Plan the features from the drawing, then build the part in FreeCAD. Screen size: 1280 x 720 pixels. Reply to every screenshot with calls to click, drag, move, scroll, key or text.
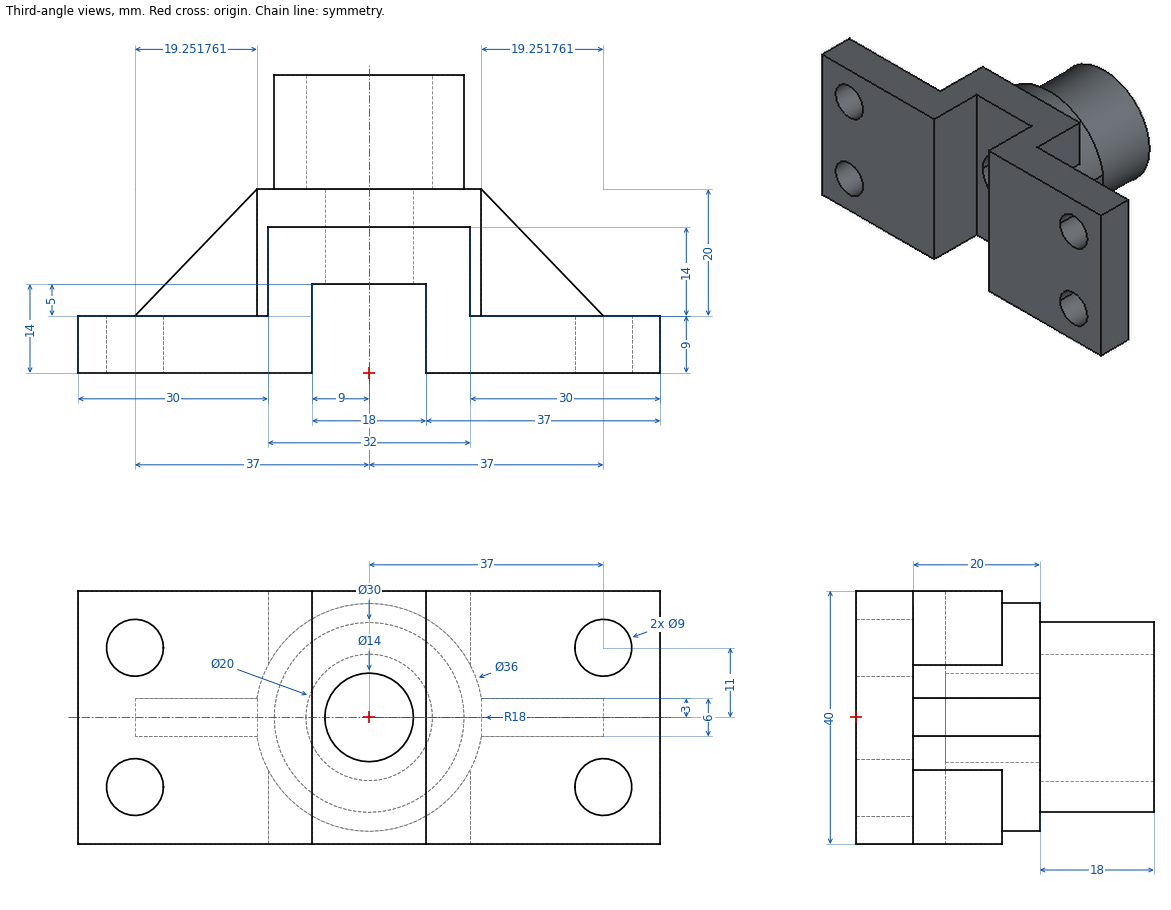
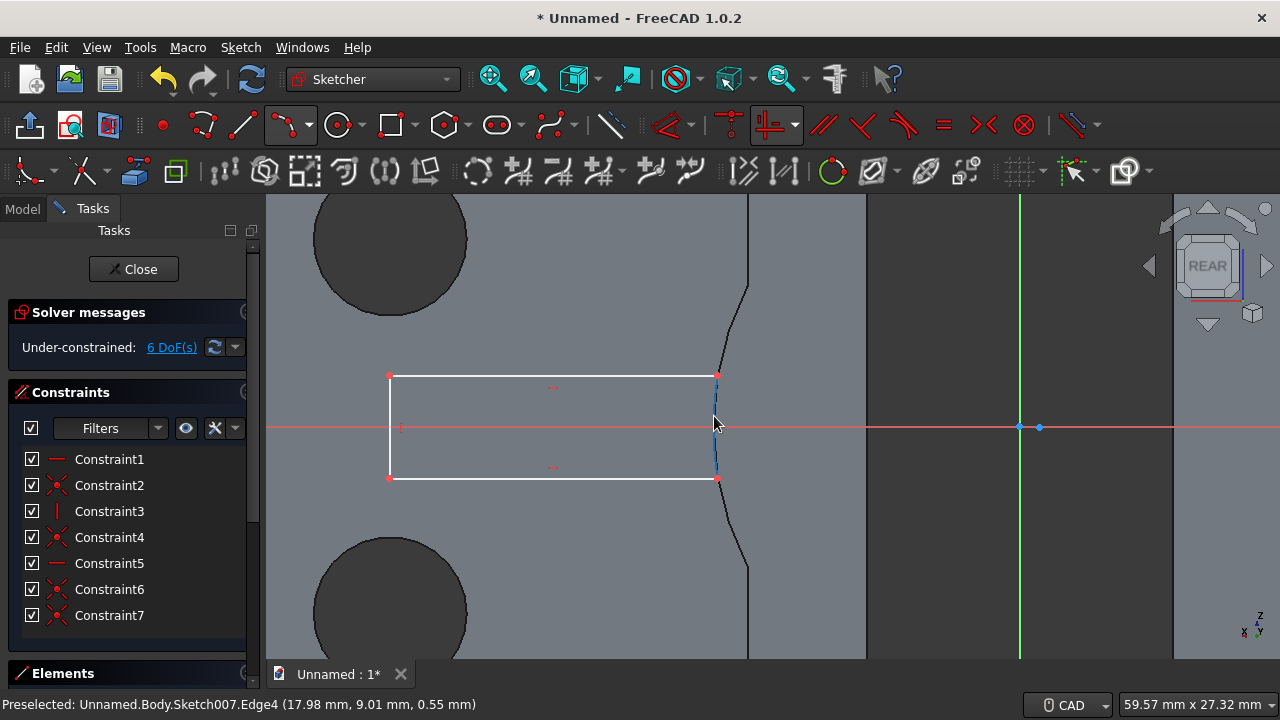
drag(1010, 416, 1049, 438)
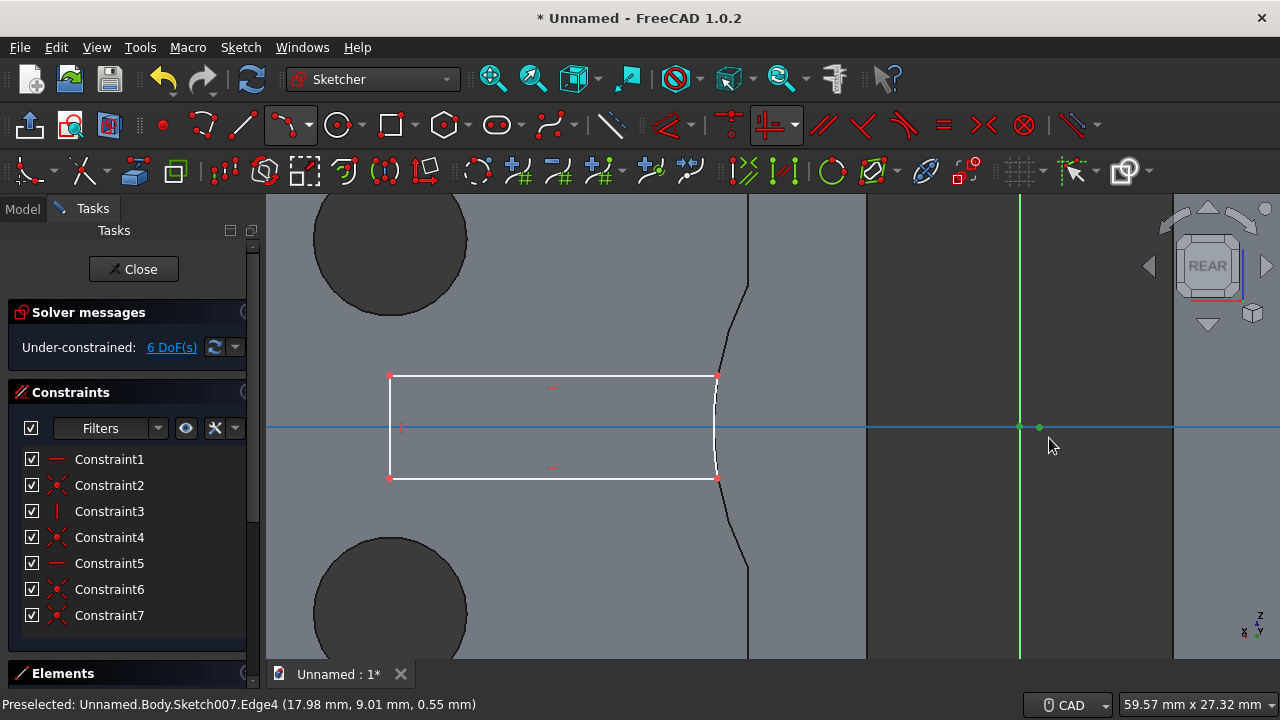
key(c)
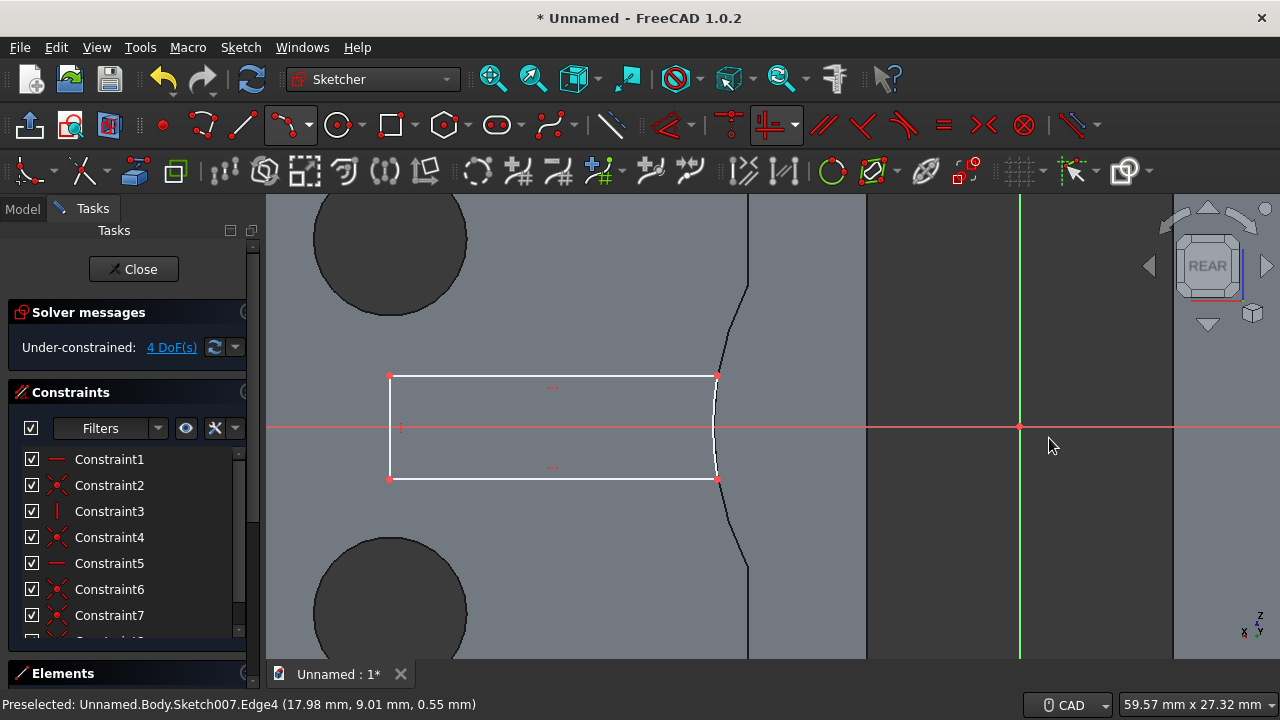
click(666, 126)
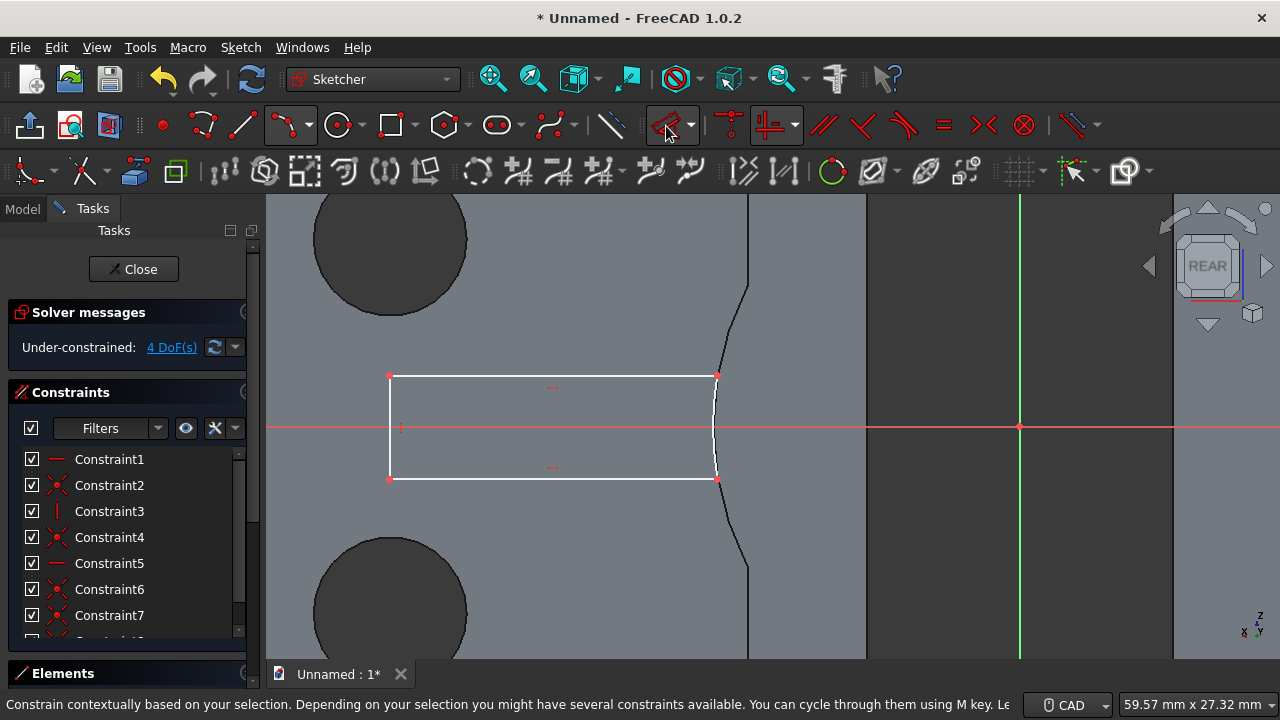
click(714, 407)
click(682, 405)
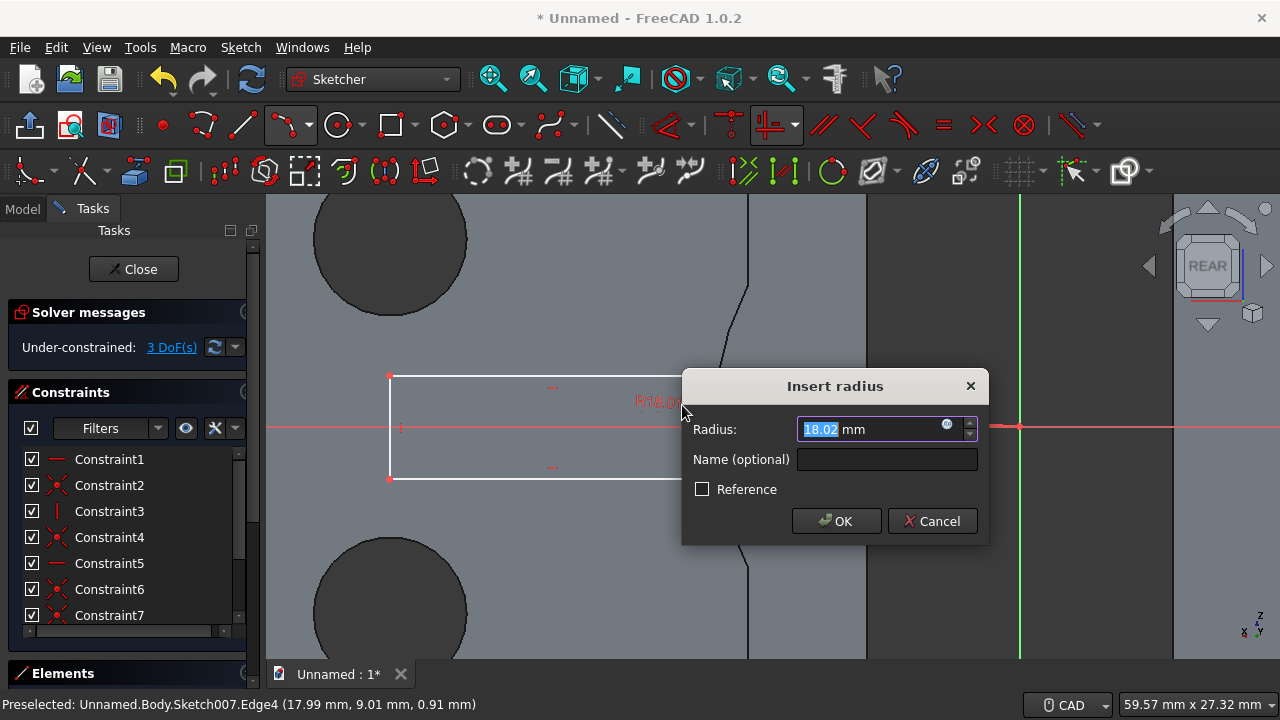
text(18)
key(Return)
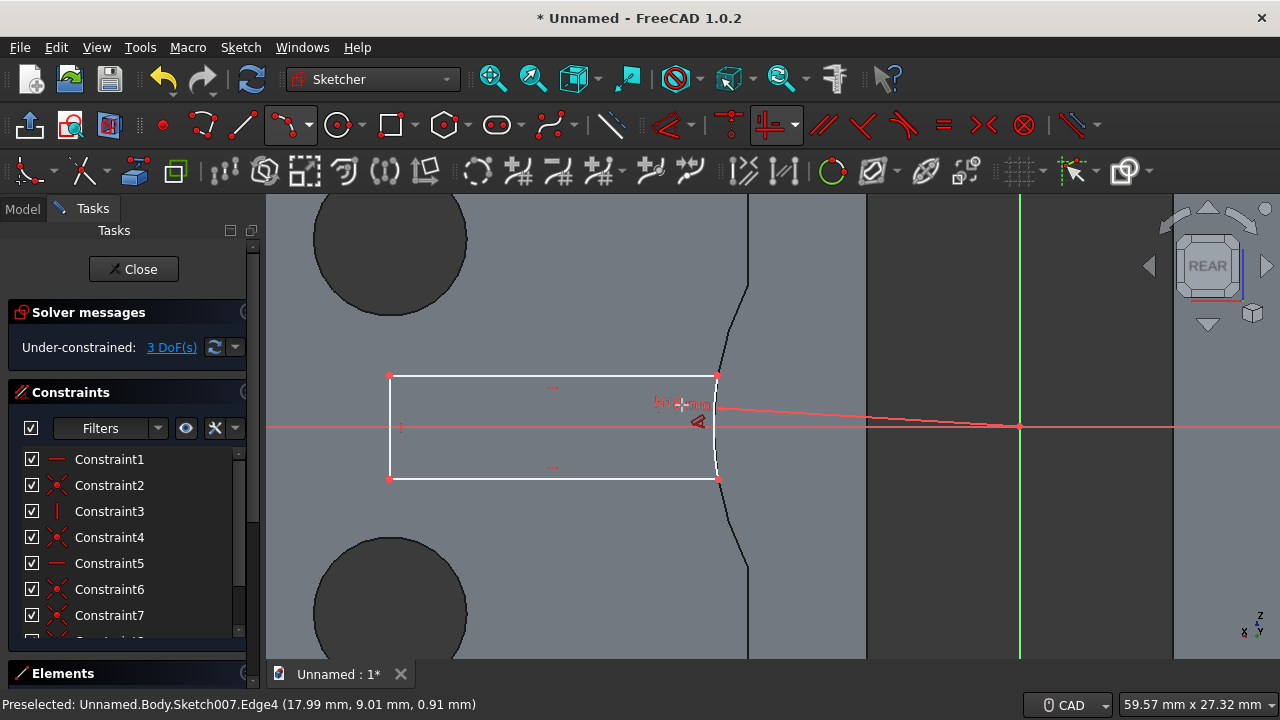
click(390, 407)
click(356, 404)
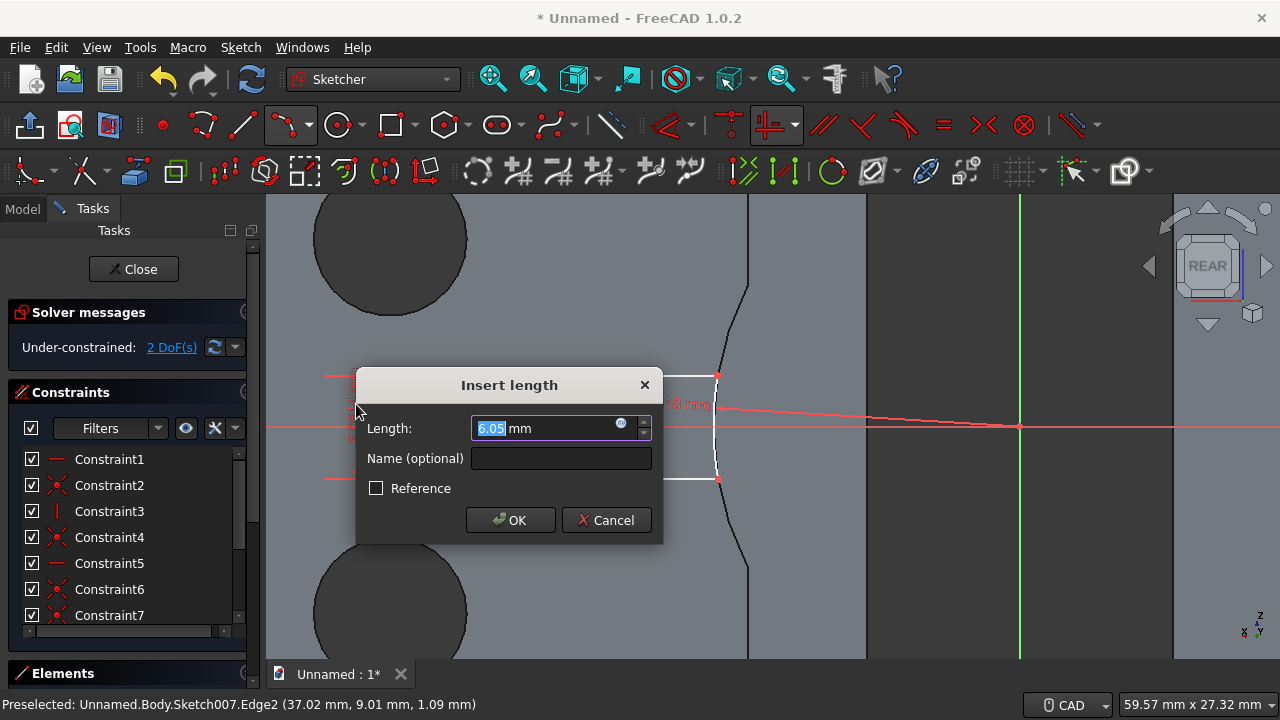
text(6)
key(Return)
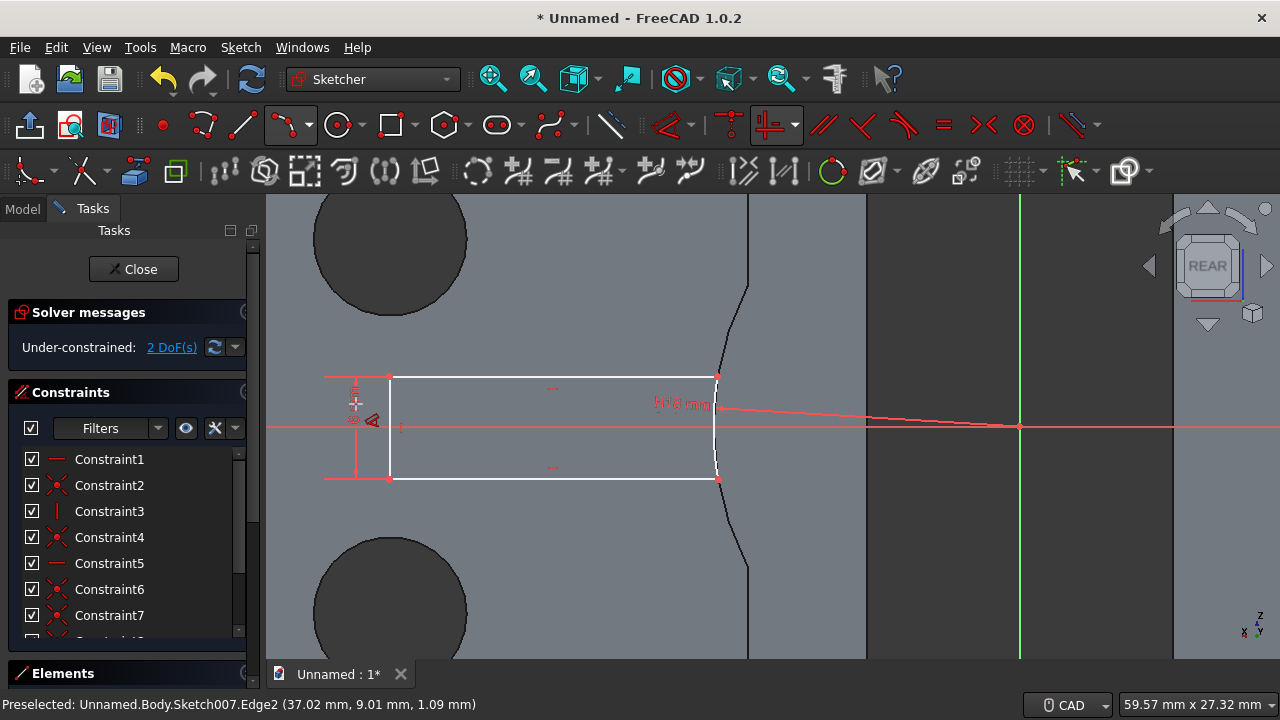
click(718, 377)
click(1054, 402)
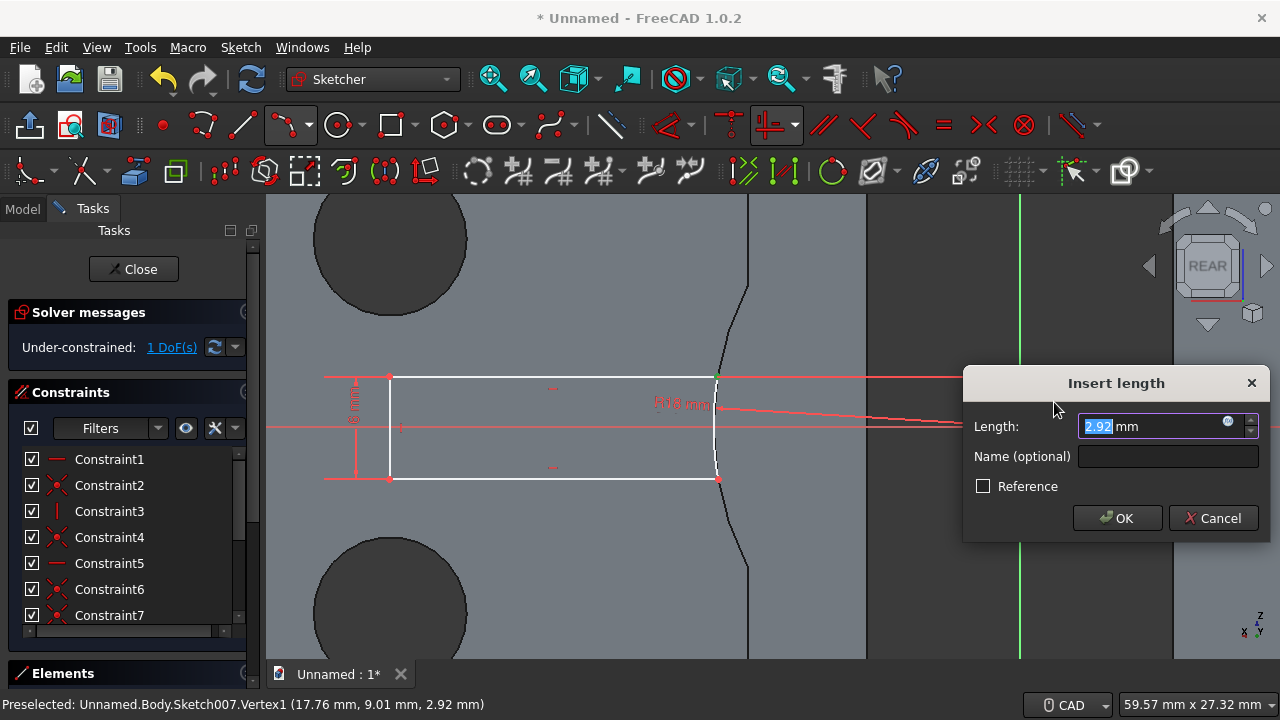
text(3)
key(Return)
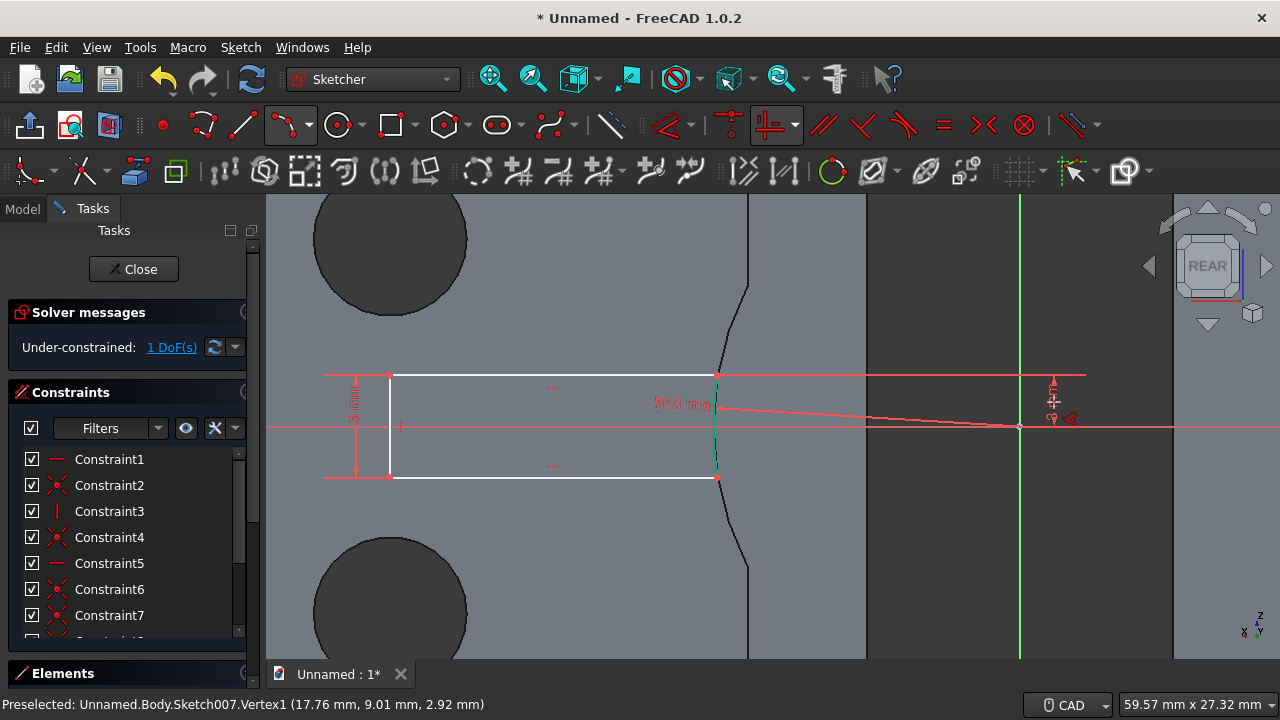
click(390, 375)
click(705, 341)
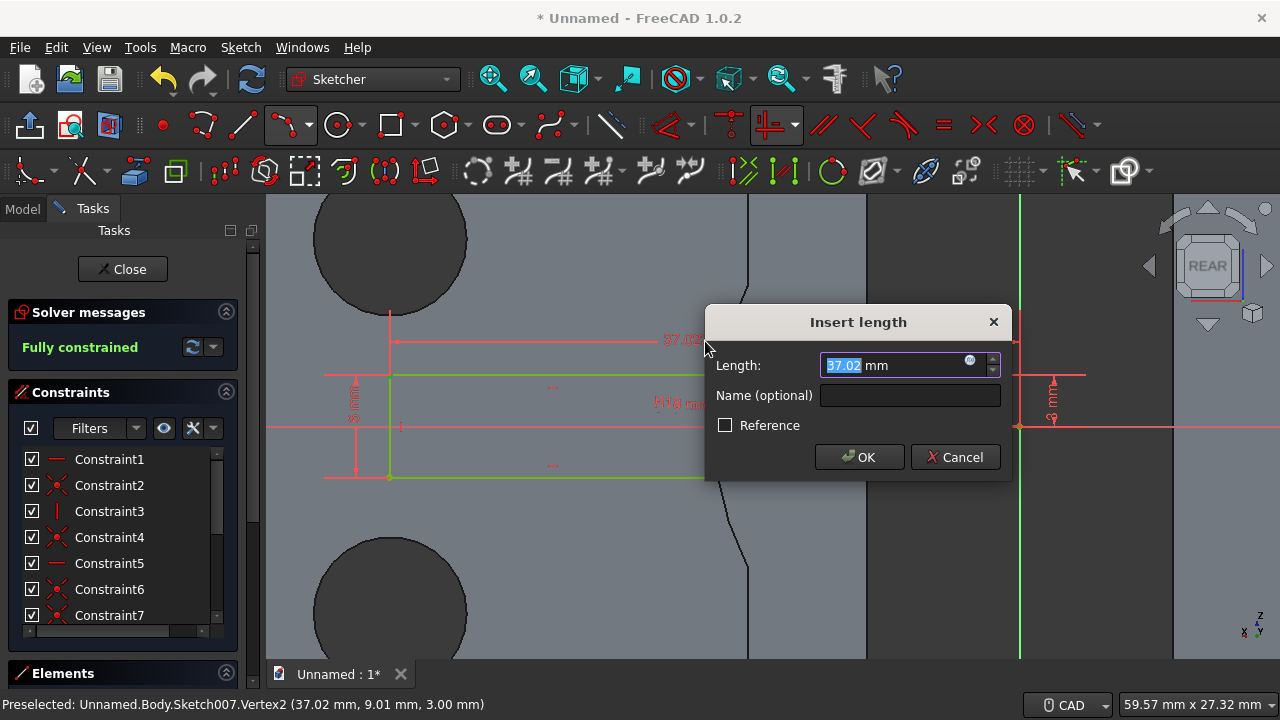
text(37)
key(Return)
key(Escape)